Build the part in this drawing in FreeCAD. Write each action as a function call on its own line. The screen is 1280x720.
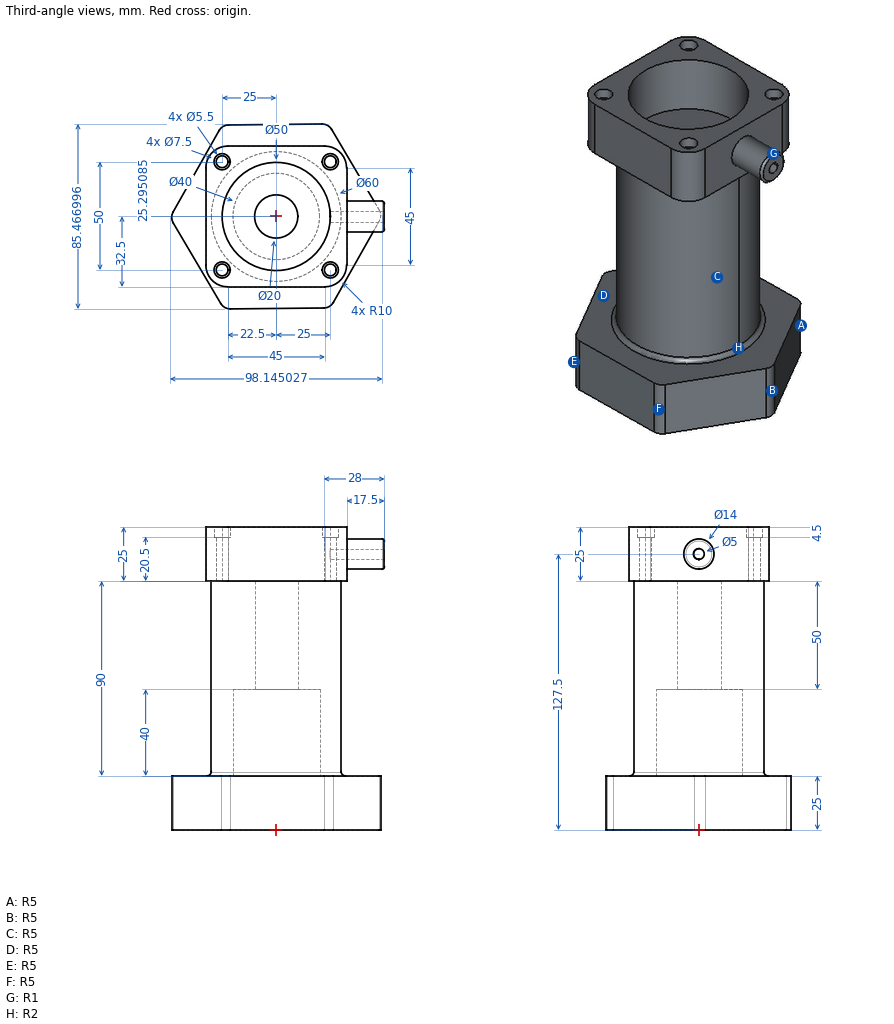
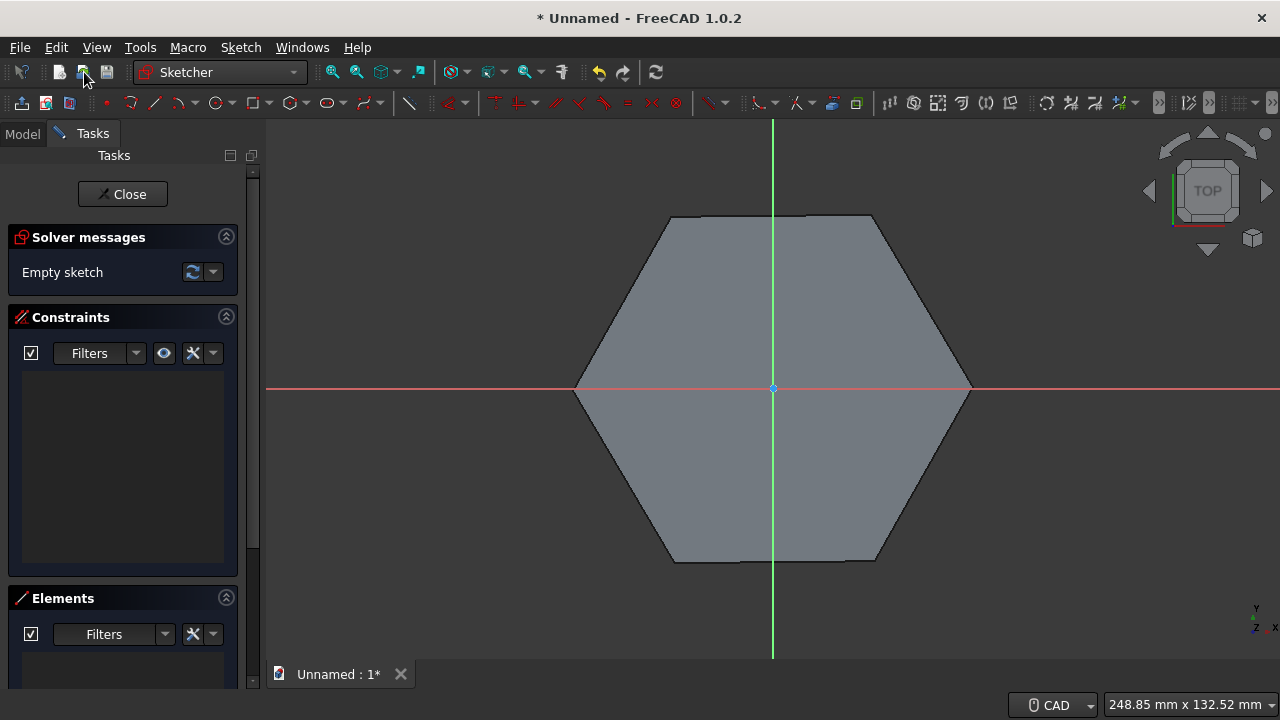
scroll(912, 389, up, 2)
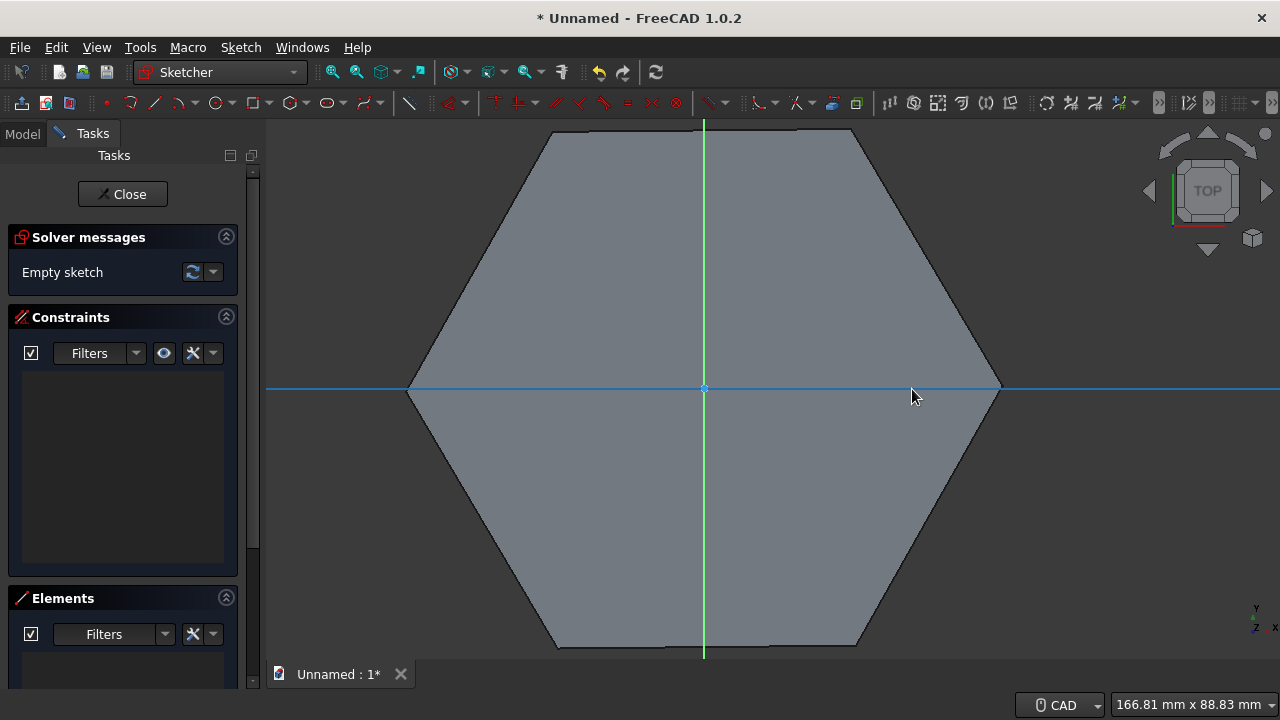
click(216, 104)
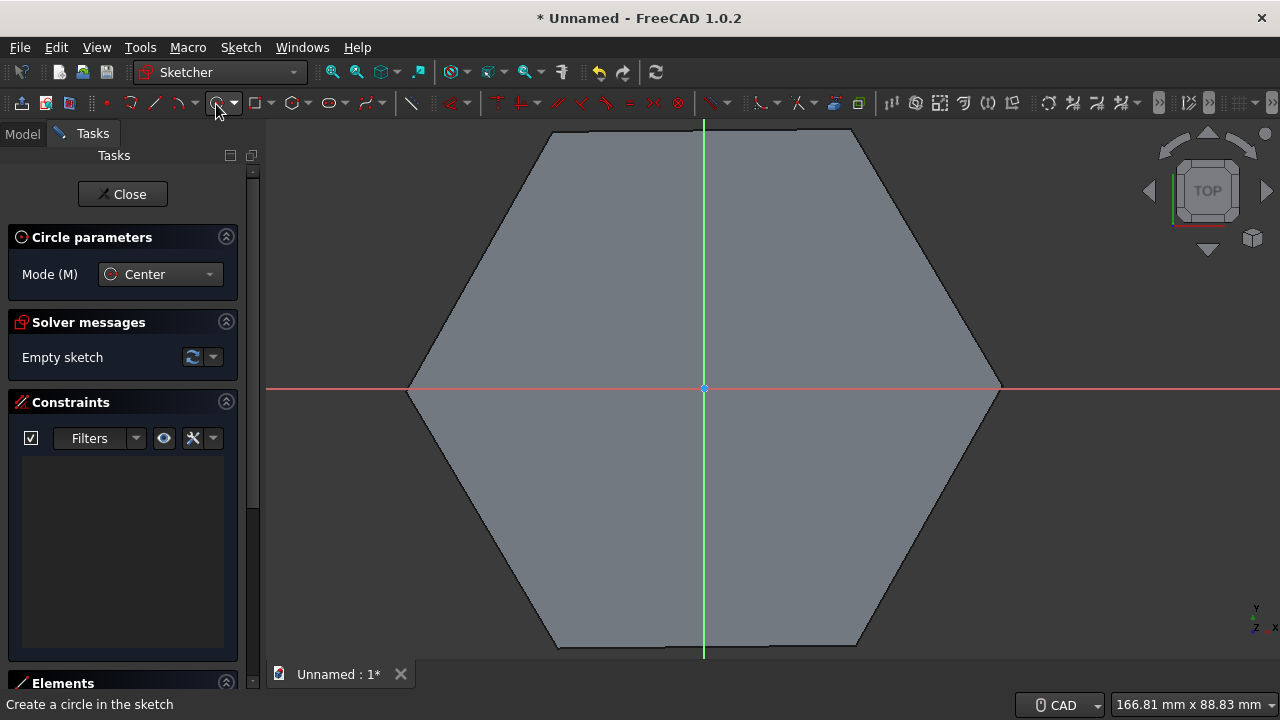
click(704, 389)
click(833, 260)
key(Escape)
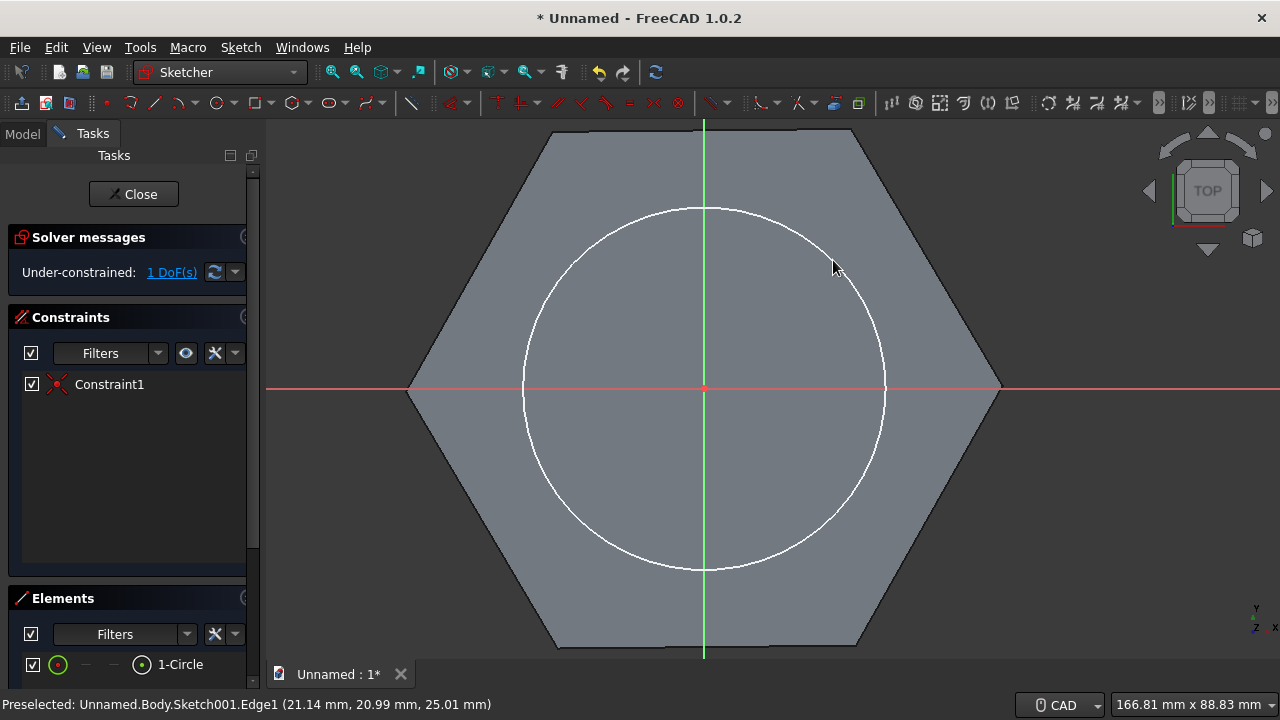
click(450, 104)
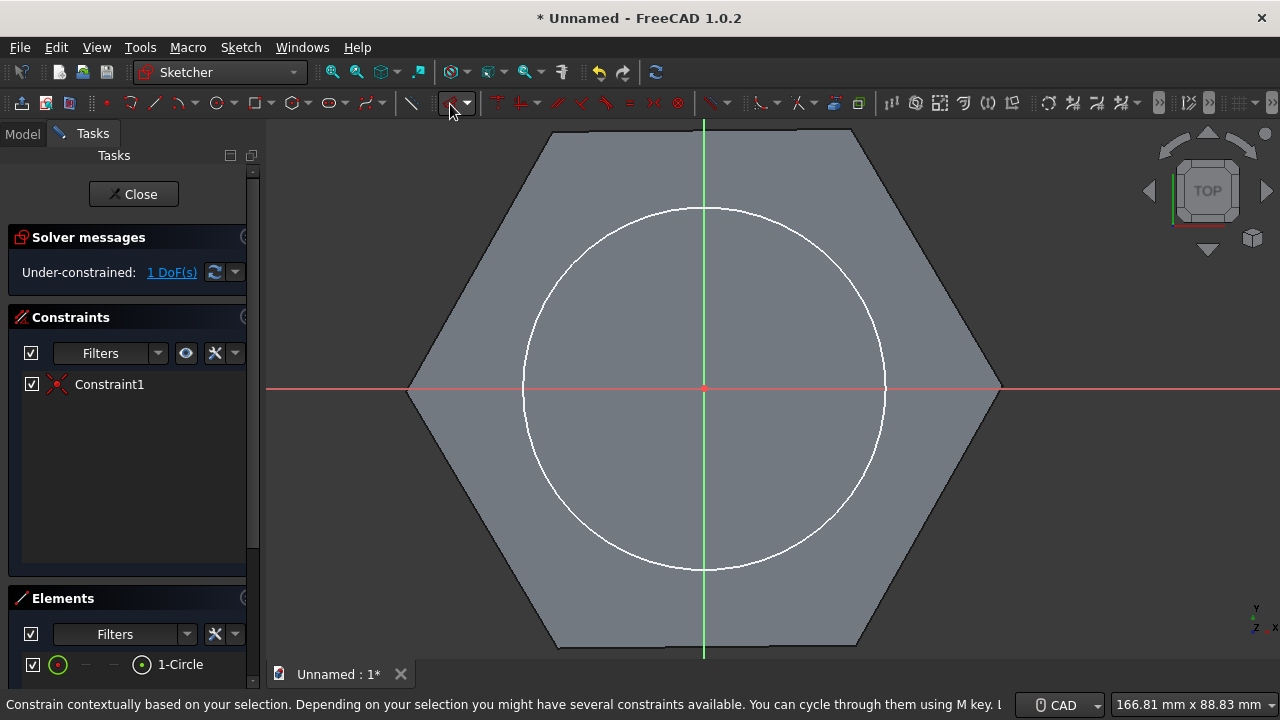
click(832, 260)
click(855, 237)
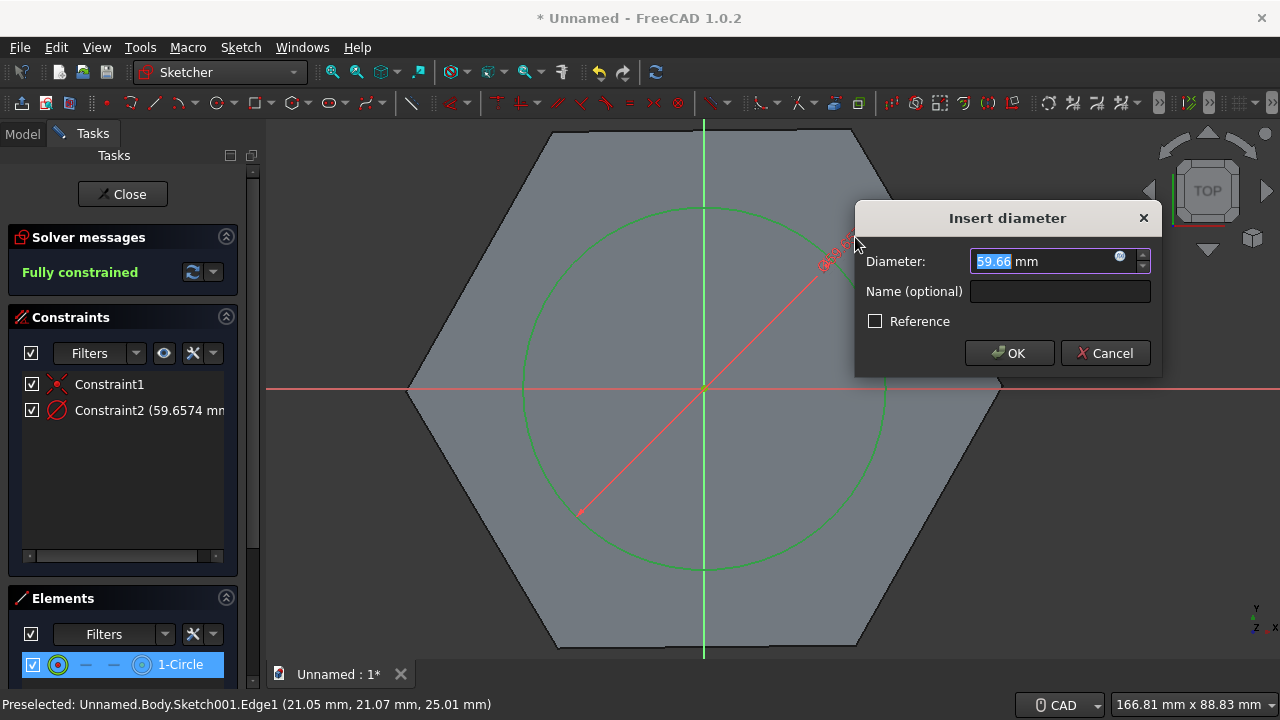
text(60)
key(Return)
key(Escape)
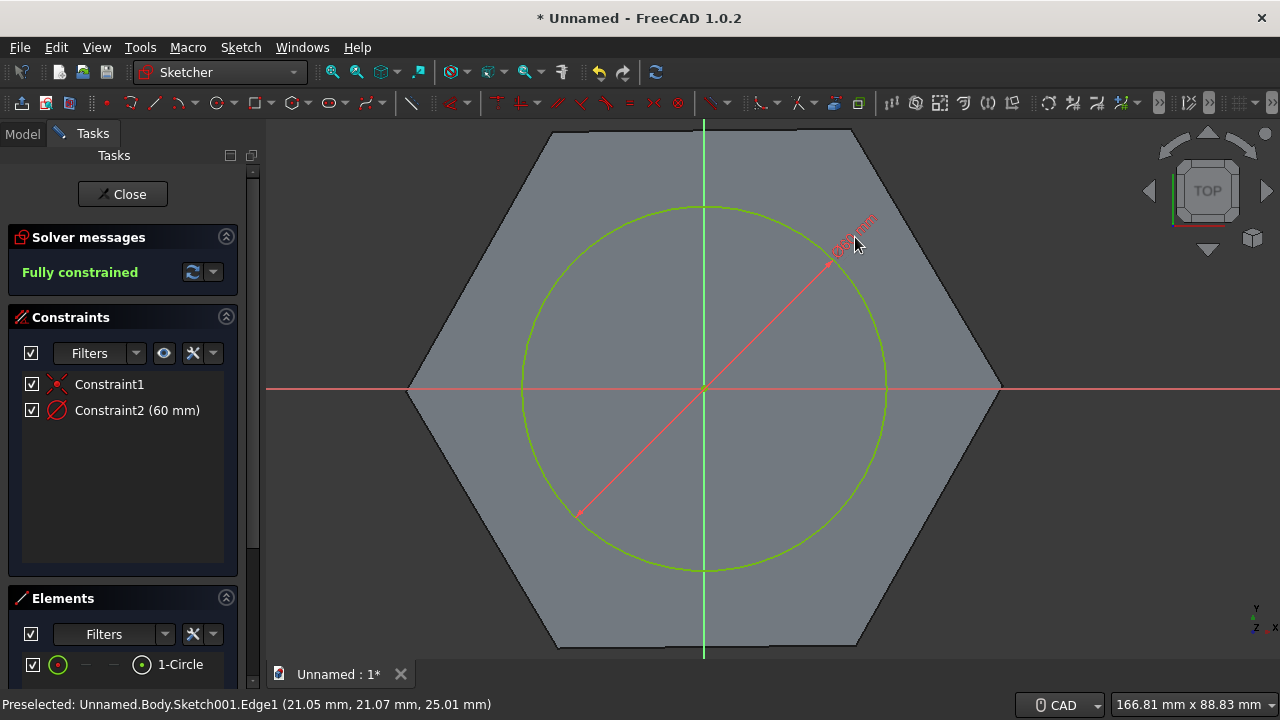
click(123, 194)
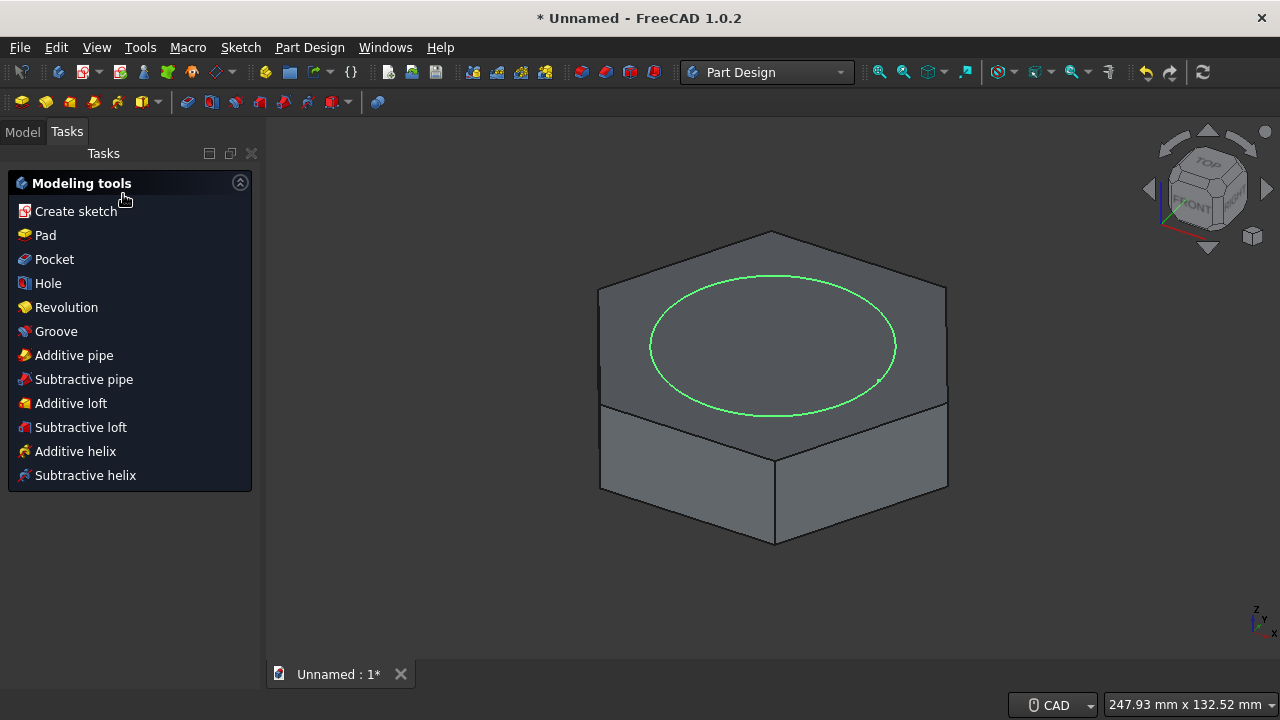
click(22, 102)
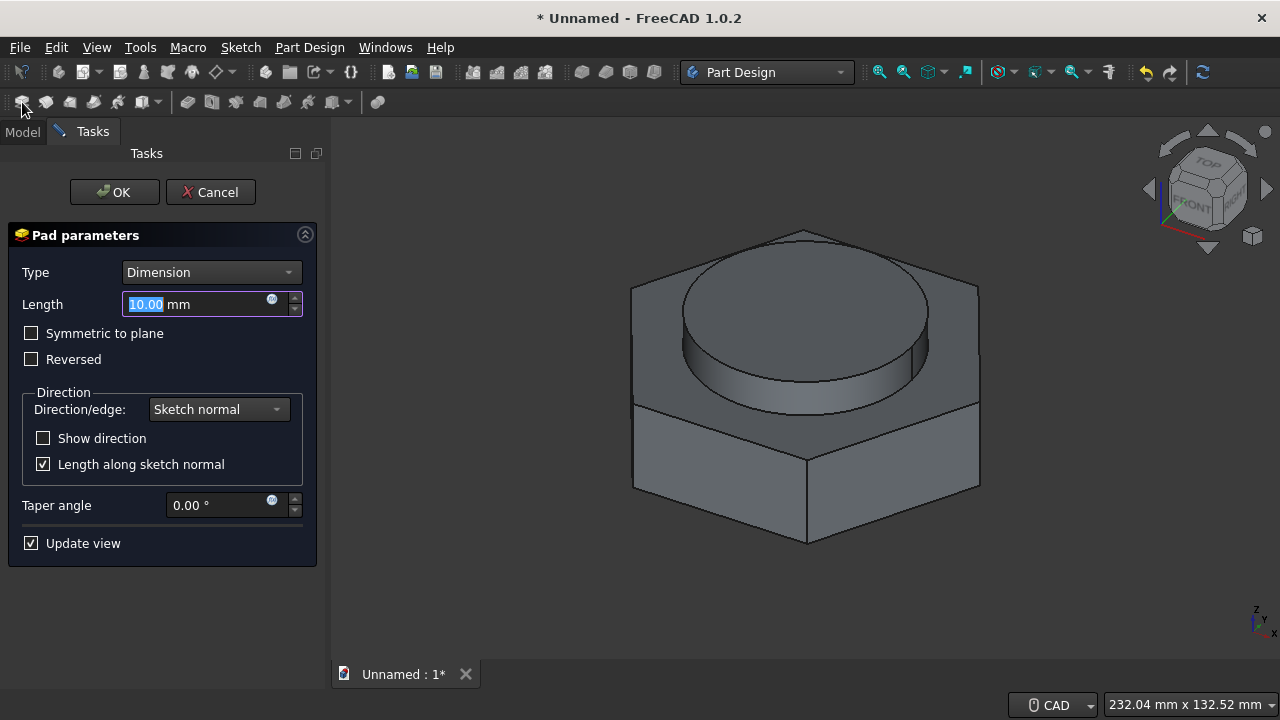
text(90)
key(Tab)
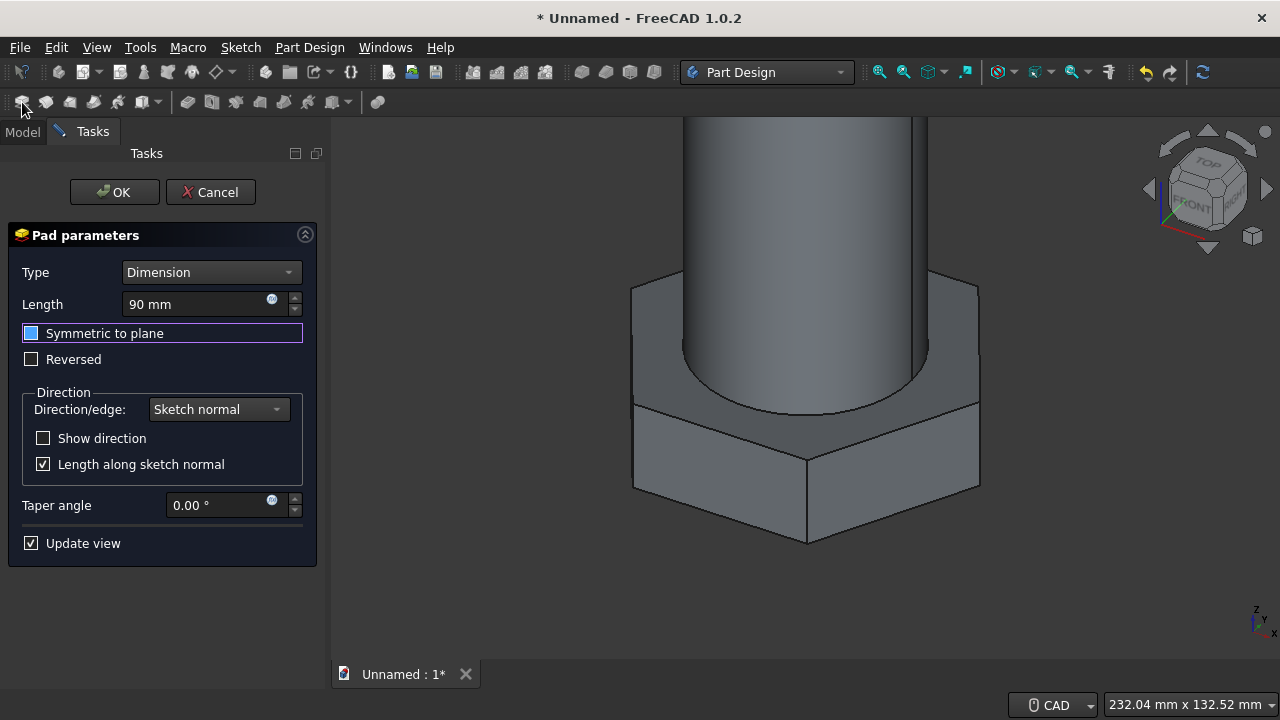
click(115, 192)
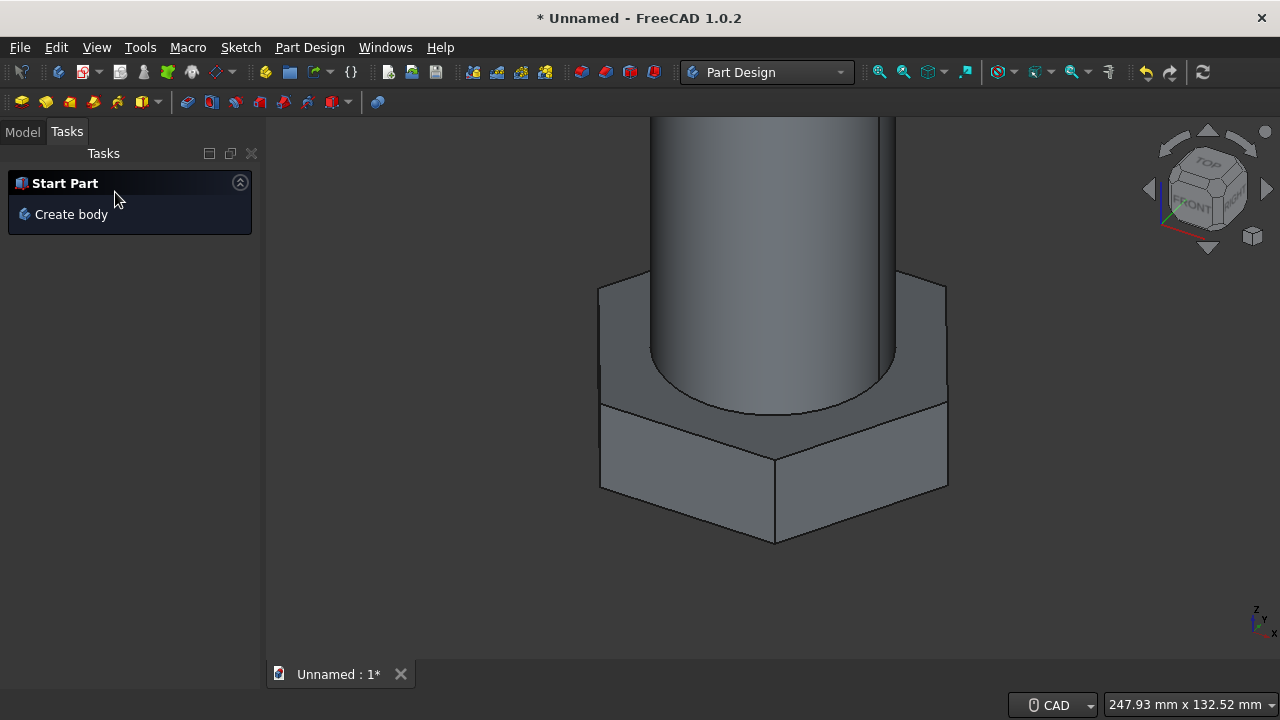
click(880, 72)